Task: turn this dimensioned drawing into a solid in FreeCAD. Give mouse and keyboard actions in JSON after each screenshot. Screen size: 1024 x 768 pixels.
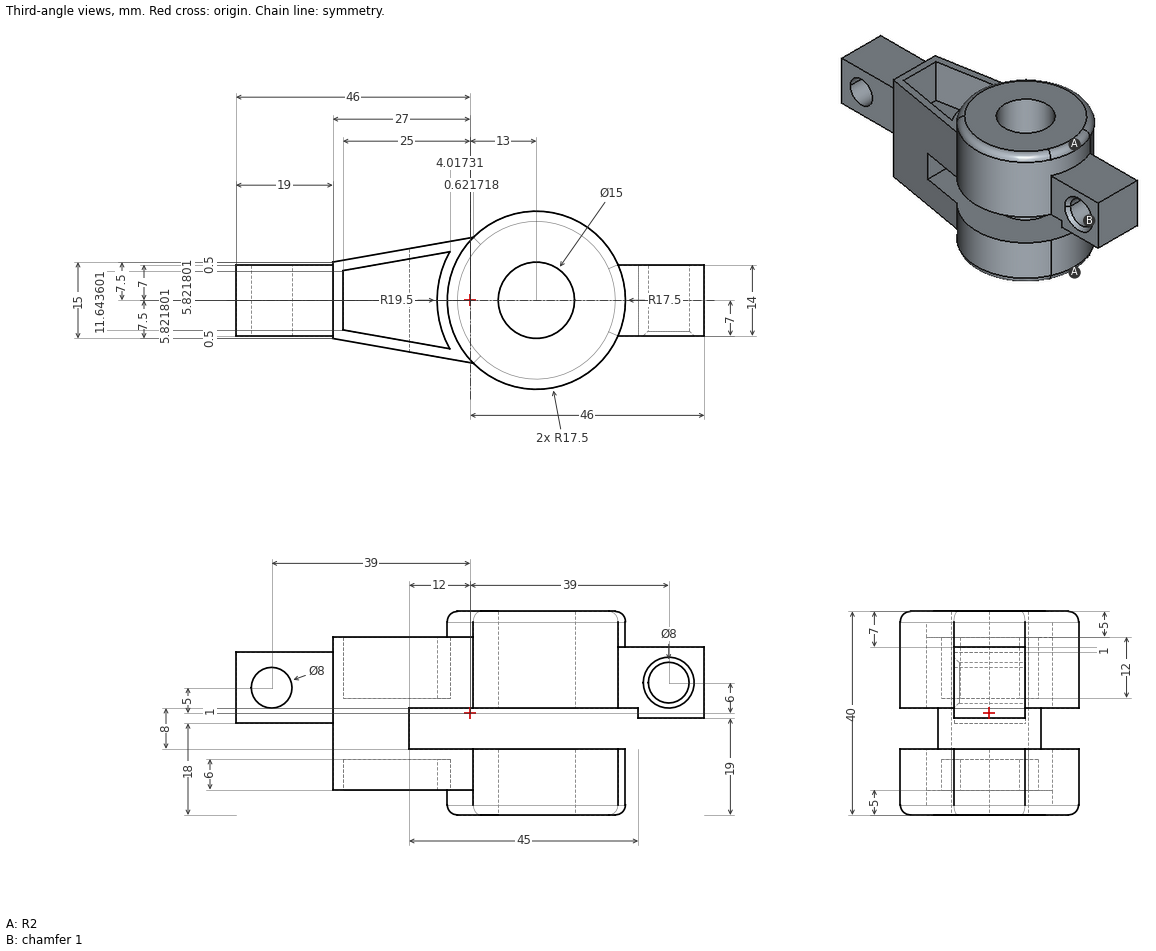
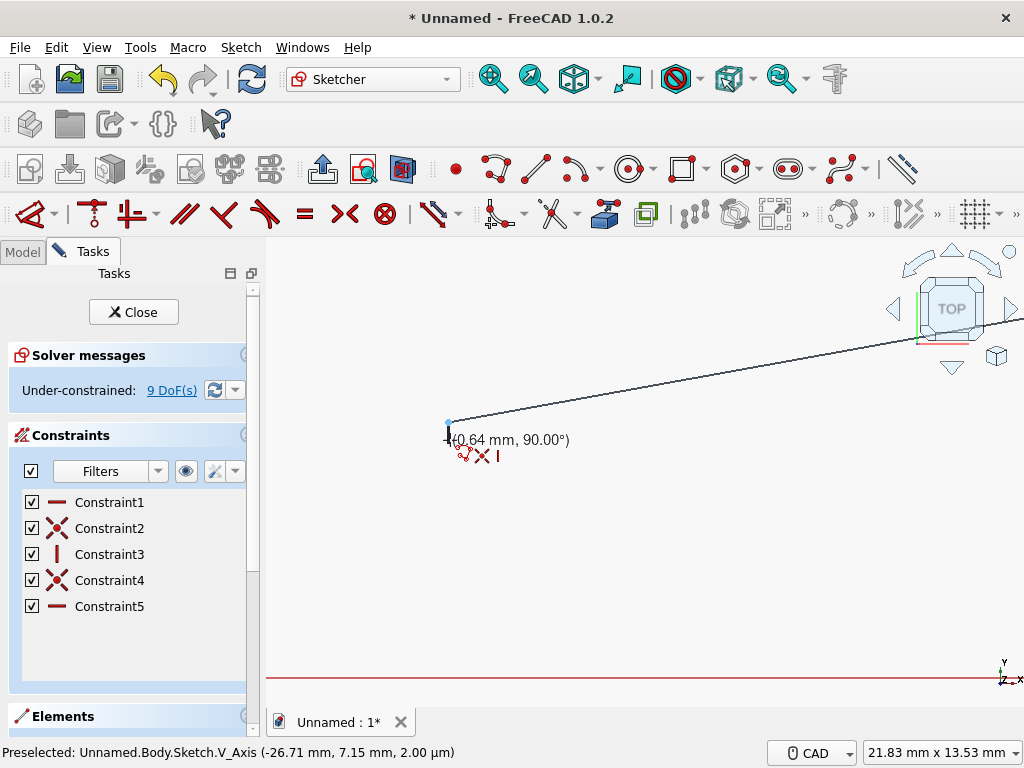
{"action": "left_click", "coordinate": [448, 435]}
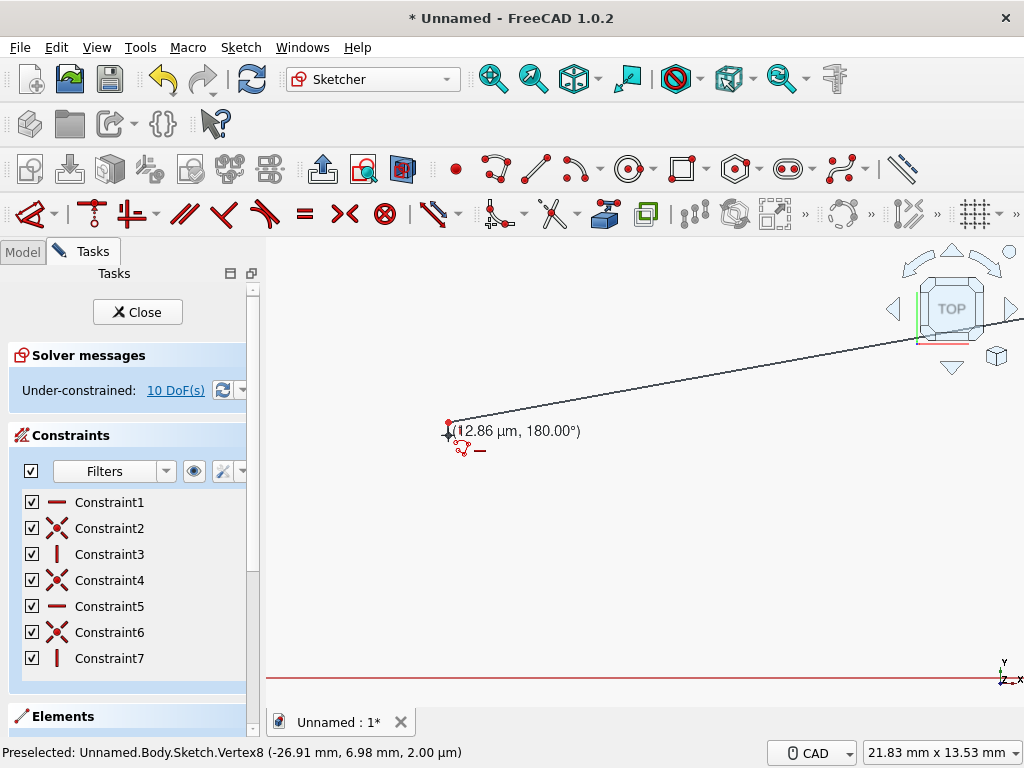
{"action": "scroll", "coordinate": [450, 440], "scroll_direction": "down", "scroll_amount": 10}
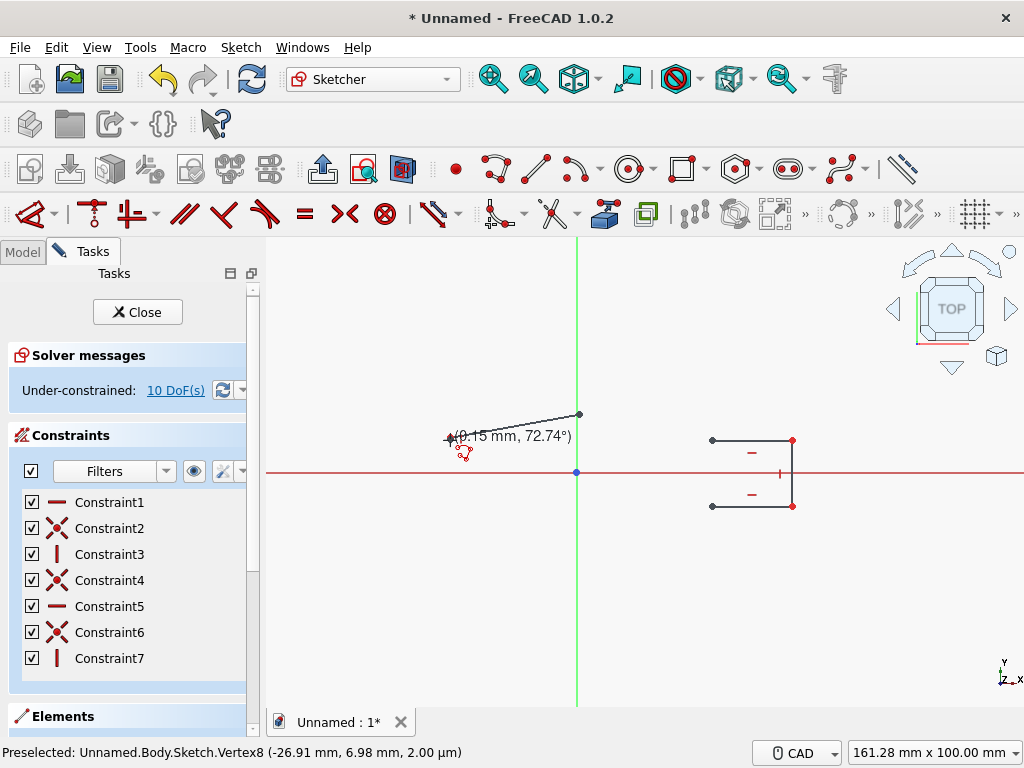
{"action": "left_click", "coordinate": [360, 440]}
{"action": "left_click", "coordinate": [360, 506]}
{"action": "left_click", "coordinate": [450, 506]}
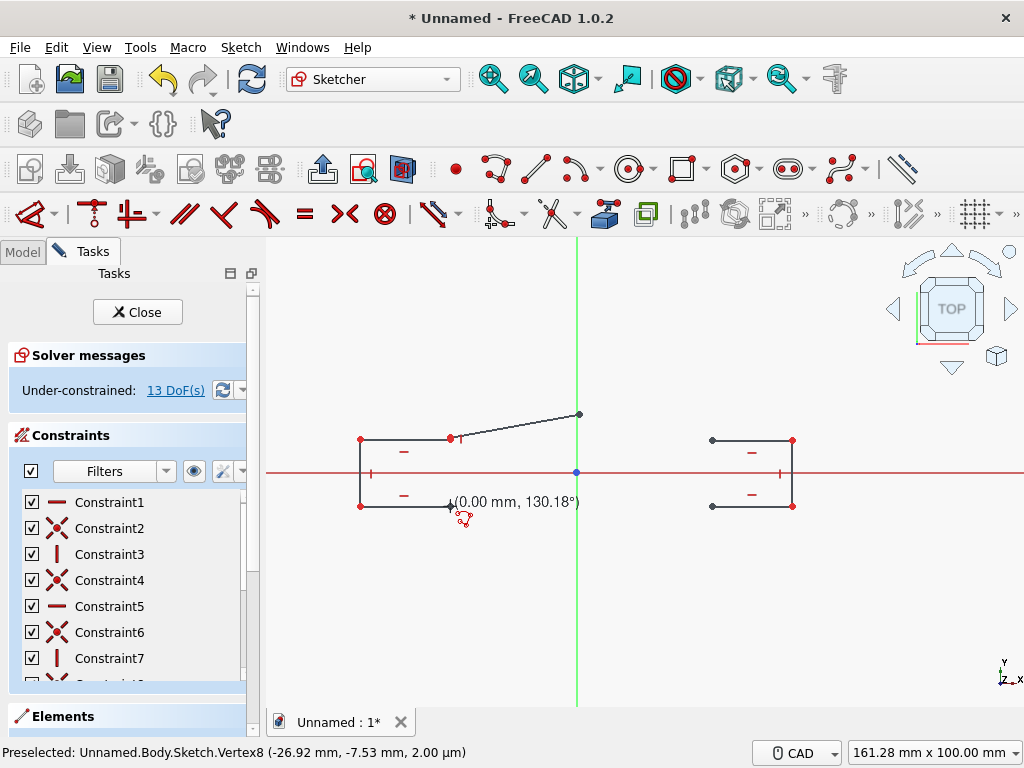
{"action": "scroll", "coordinate": [450, 508], "scroll_direction": "up", "scroll_amount": 10}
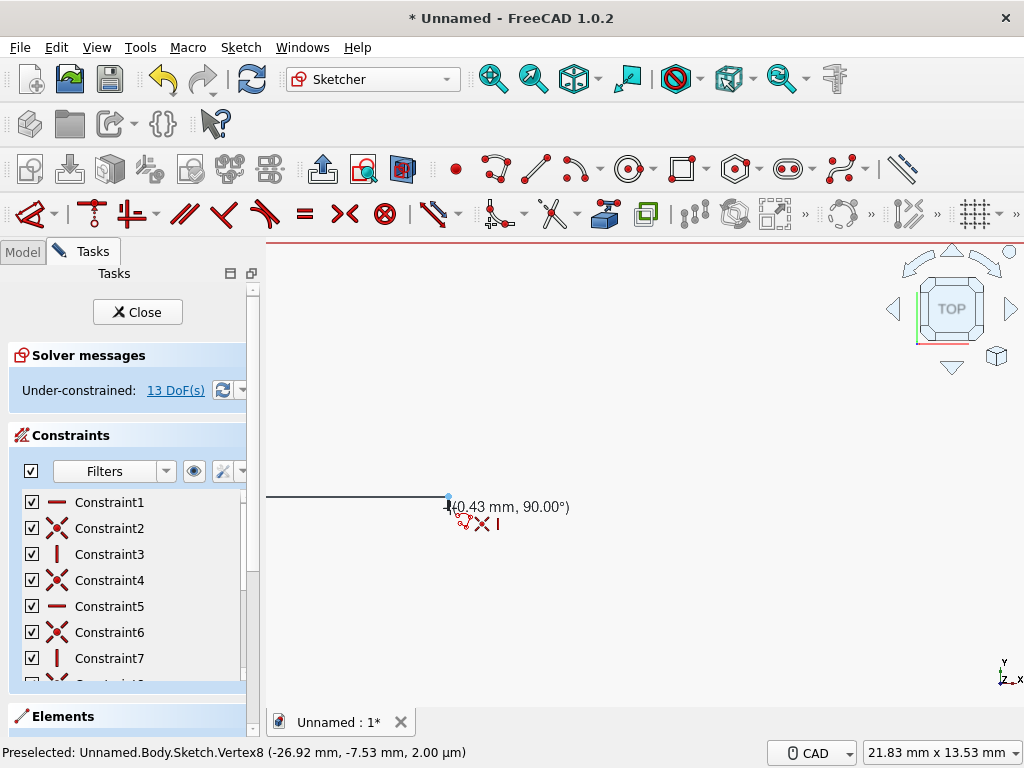
{"action": "left_click", "coordinate": [448, 503]}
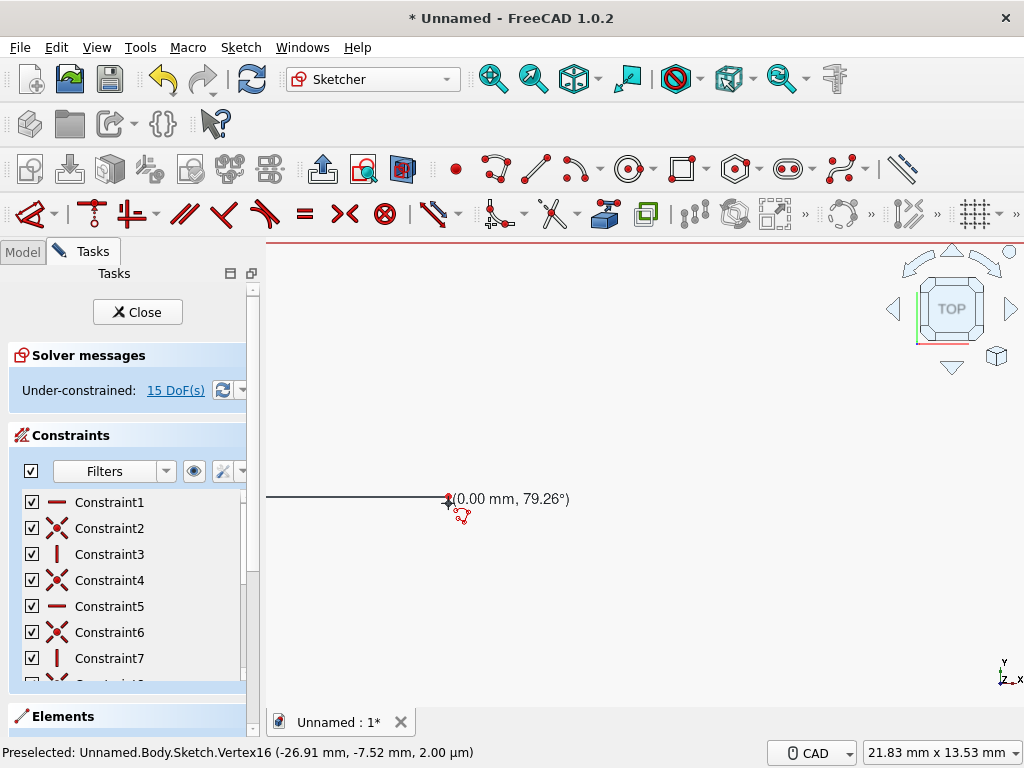
{"action": "scroll", "coordinate": [450, 508], "scroll_direction": "down", "scroll_amount": 10}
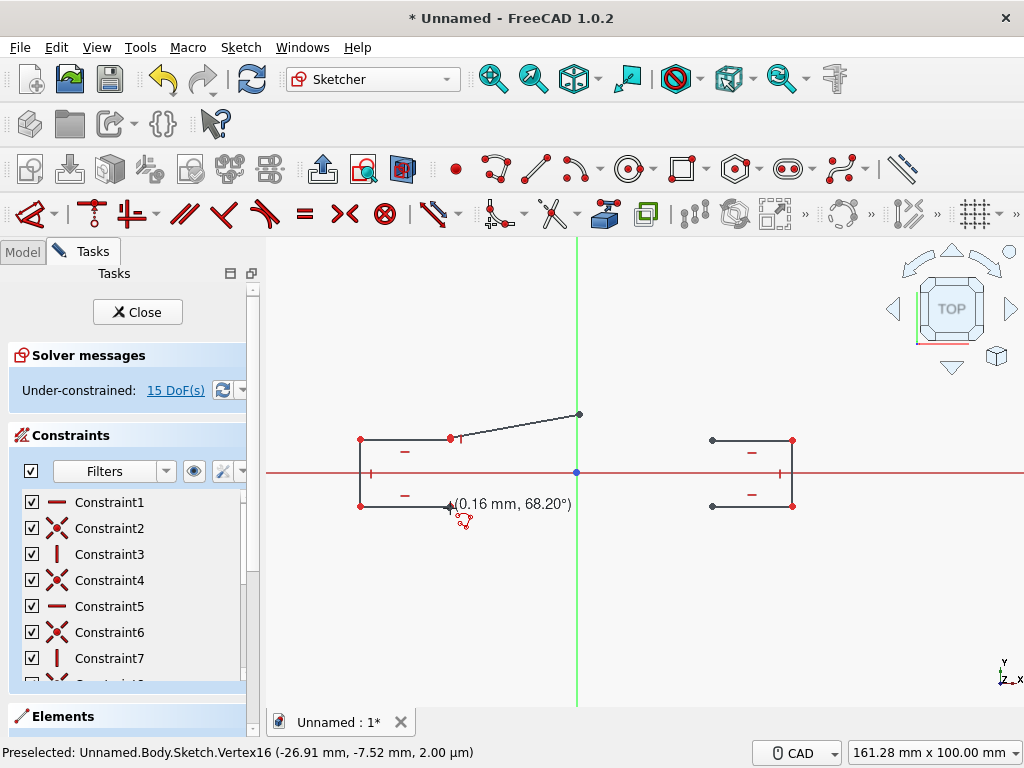
{"action": "scroll", "coordinate": [579, 531], "scroll_direction": "up", "scroll_amount": 9}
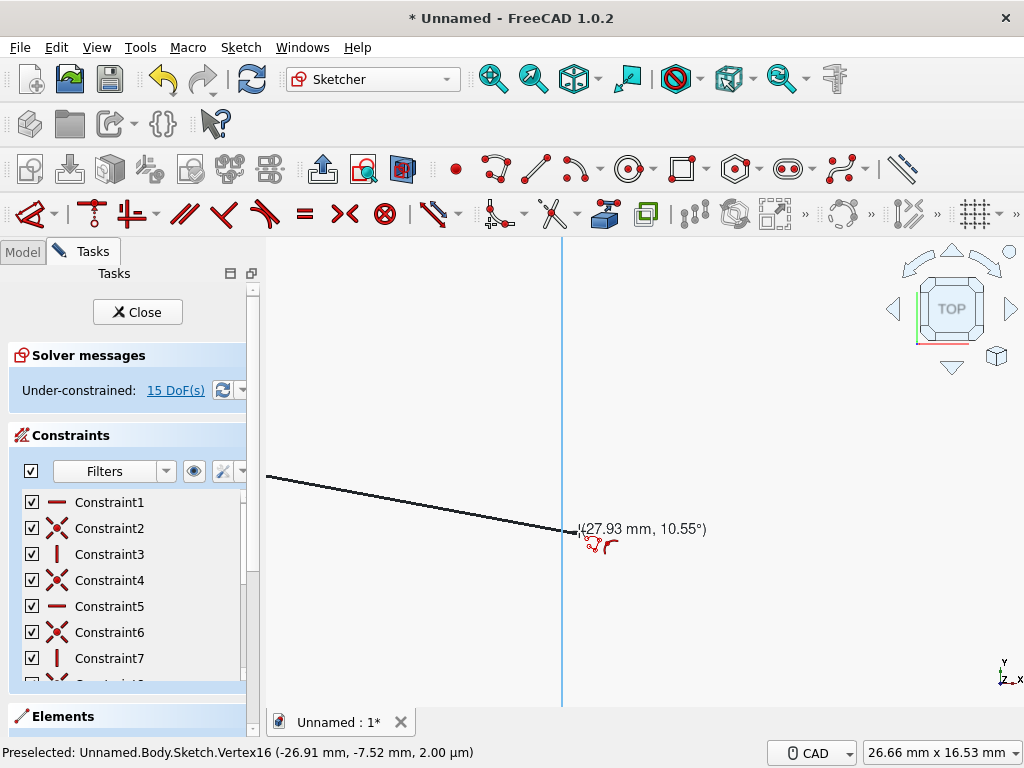
{"action": "left_click", "coordinate": [580, 526]}
{"action": "right_click", "coordinate": [580, 526]}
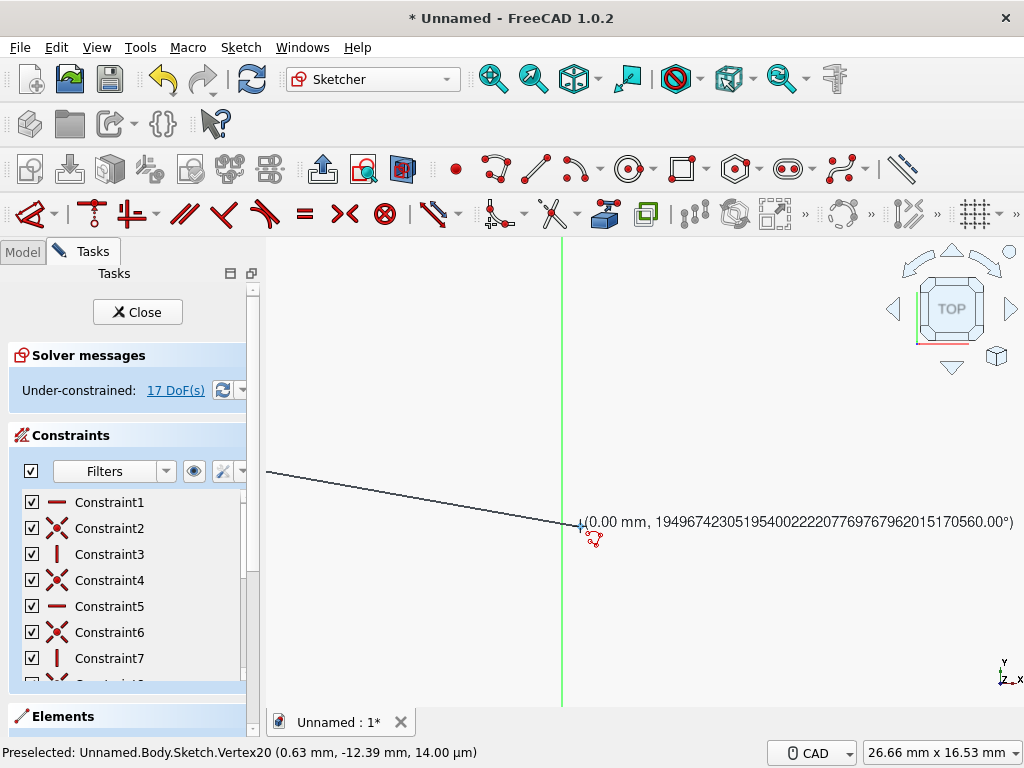
{"action": "left_click", "coordinate": [602, 170]}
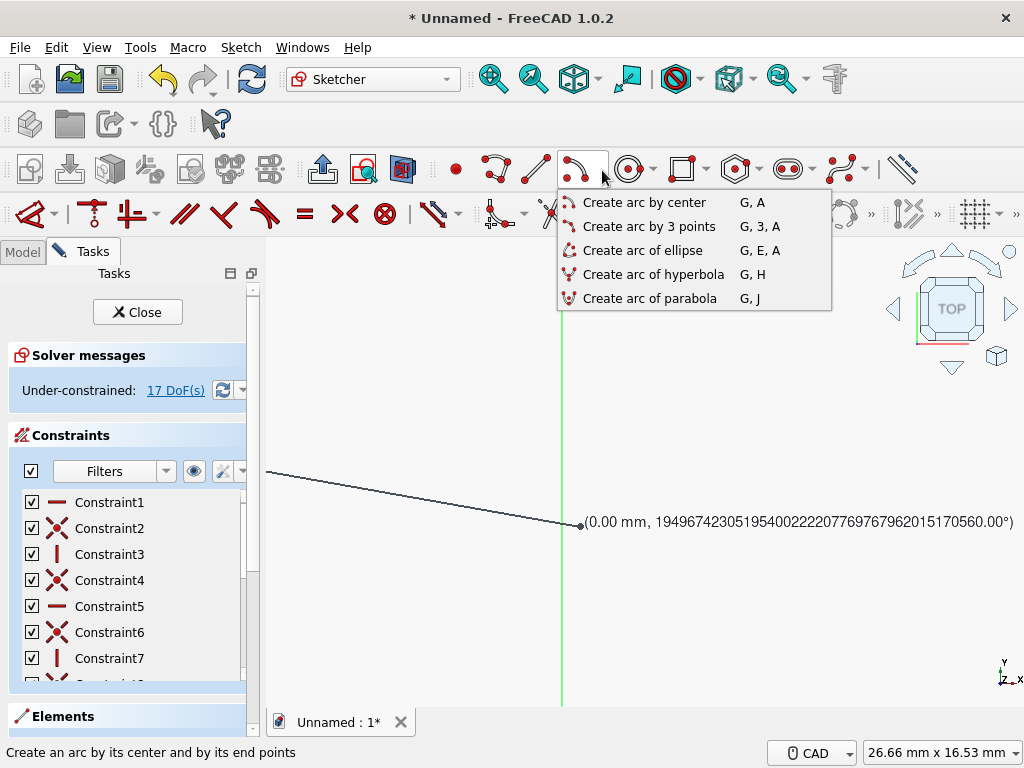
{"action": "left_click", "coordinate": [694, 226]}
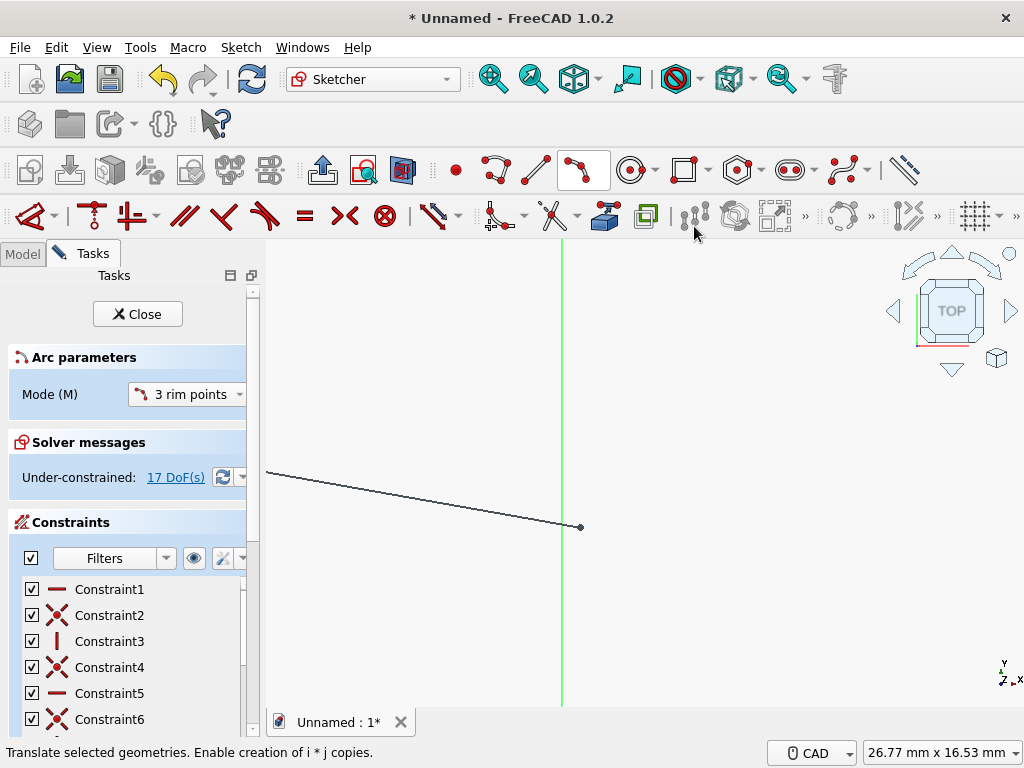
{"action": "scroll", "coordinate": [579, 532], "scroll_direction": "down", "scroll_amount": 9}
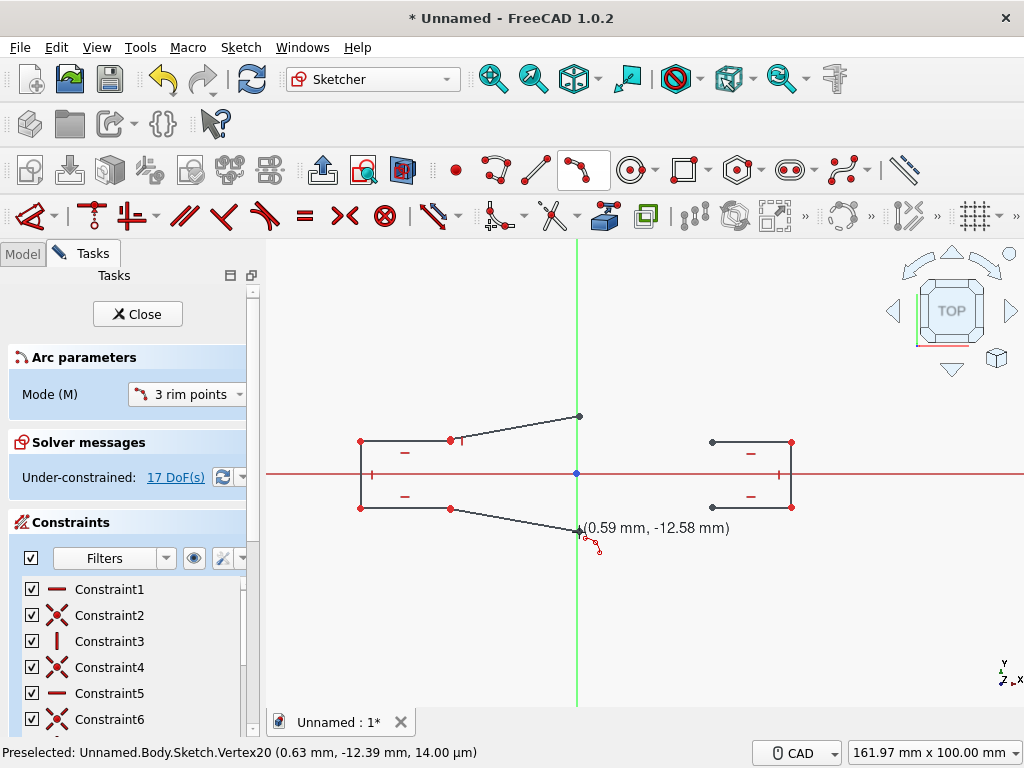
{"action": "left_click", "coordinate": [712, 442]}